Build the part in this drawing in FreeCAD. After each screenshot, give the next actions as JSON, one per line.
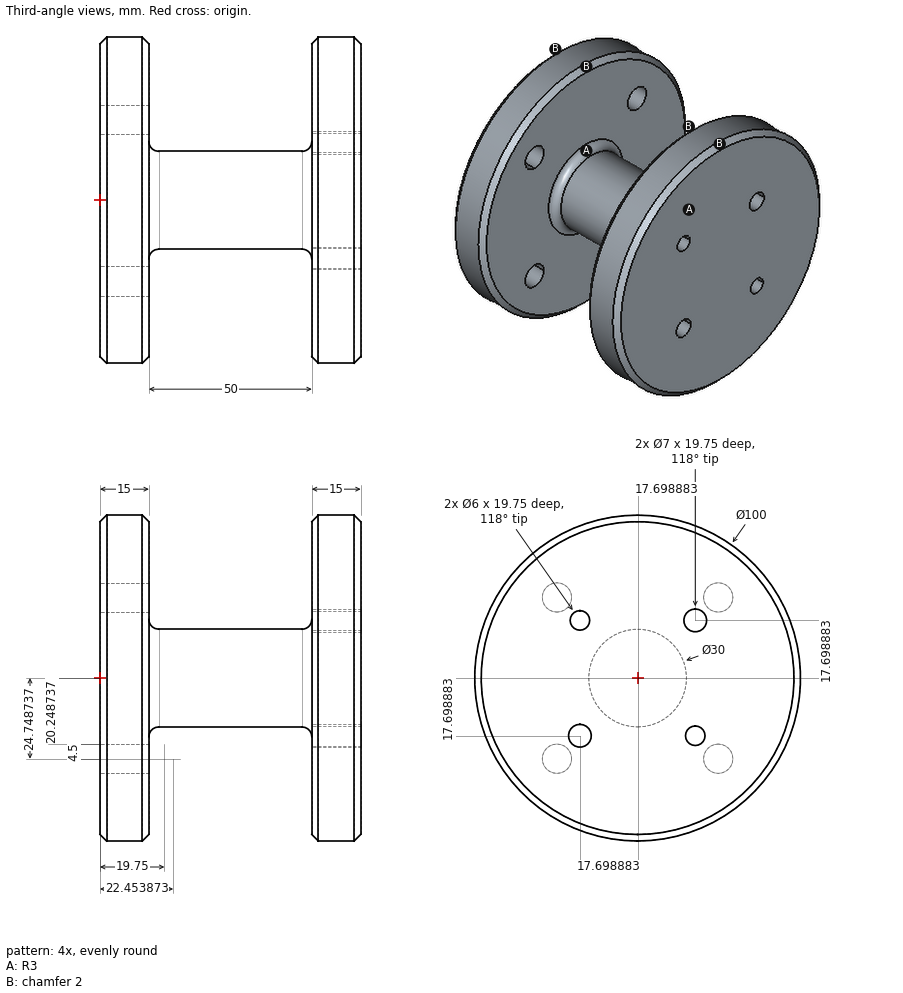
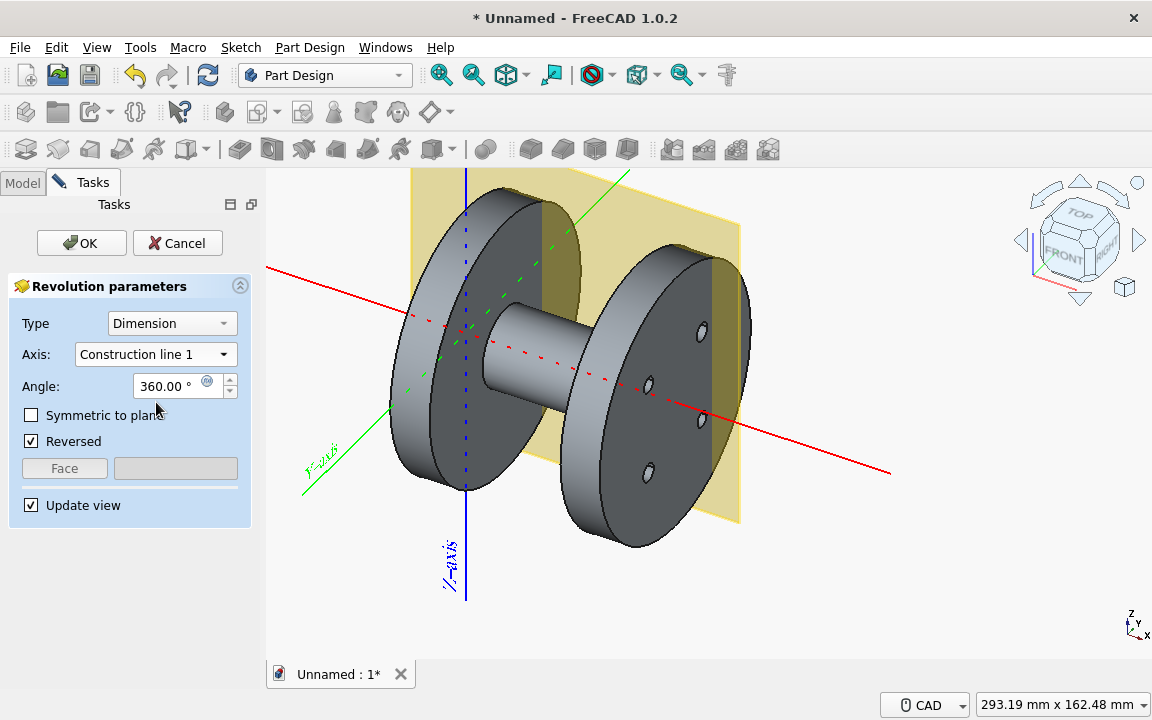
{"action": "left_click", "coordinate": [82, 243]}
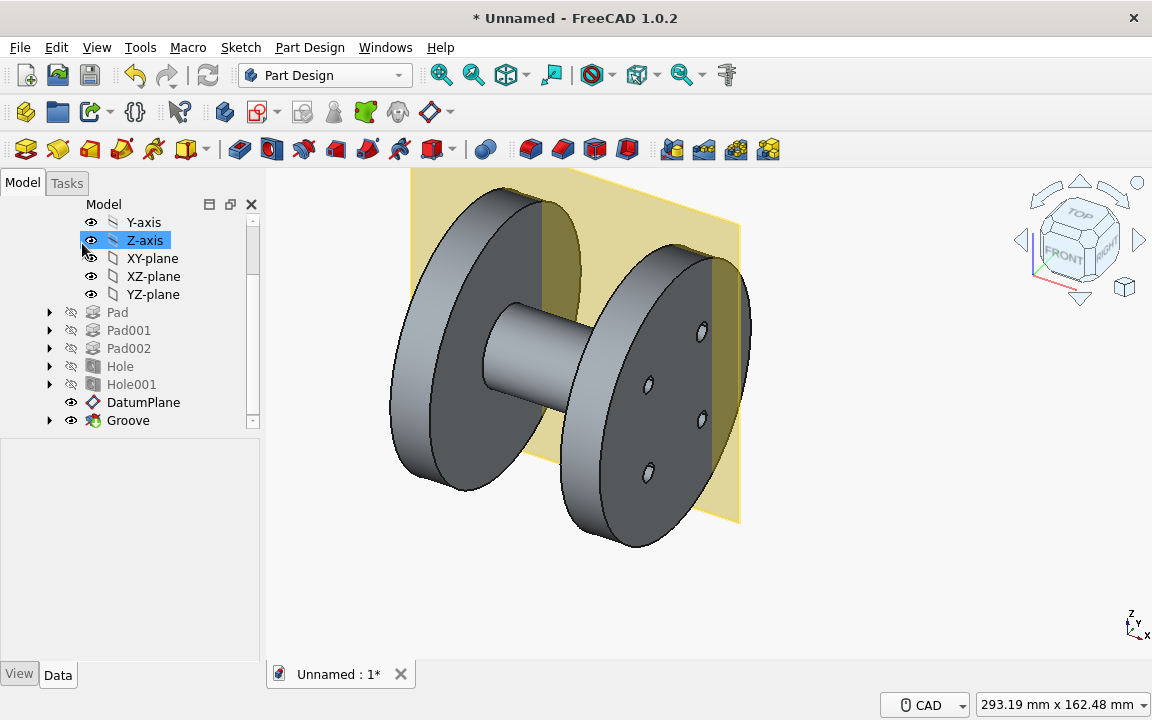
{"action": "left_click", "coordinate": [116, 402]}
{"action": "key", "text": "space"}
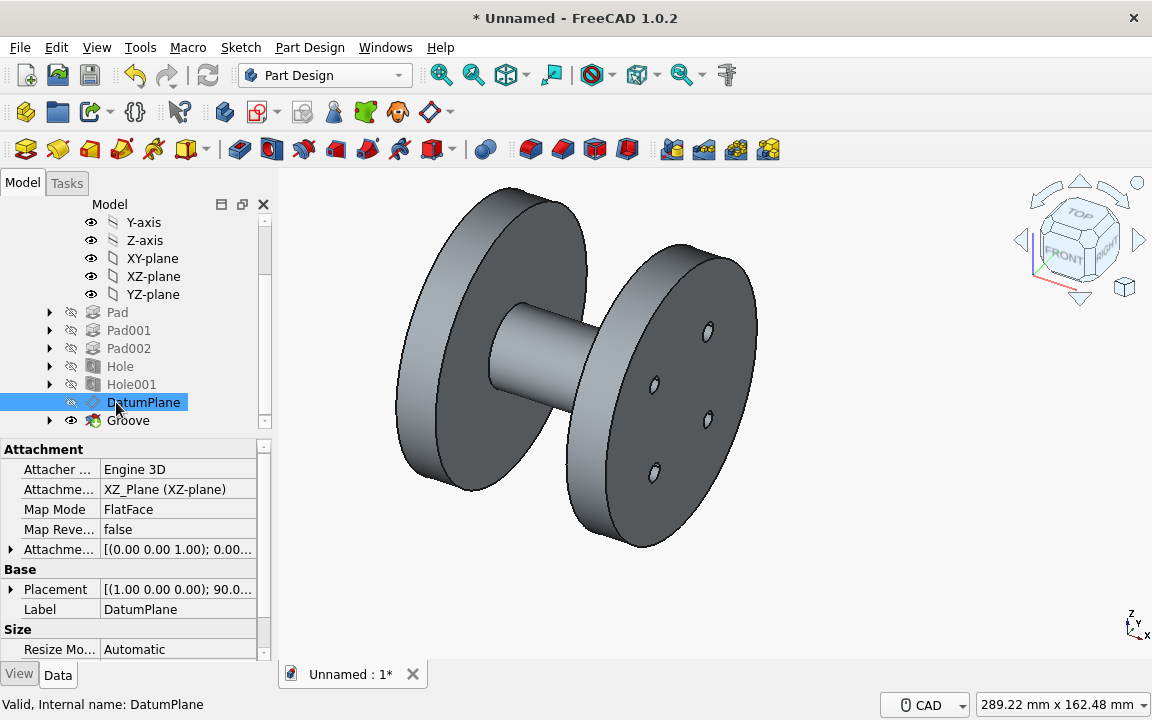
{"action": "left_click", "coordinate": [442, 76]}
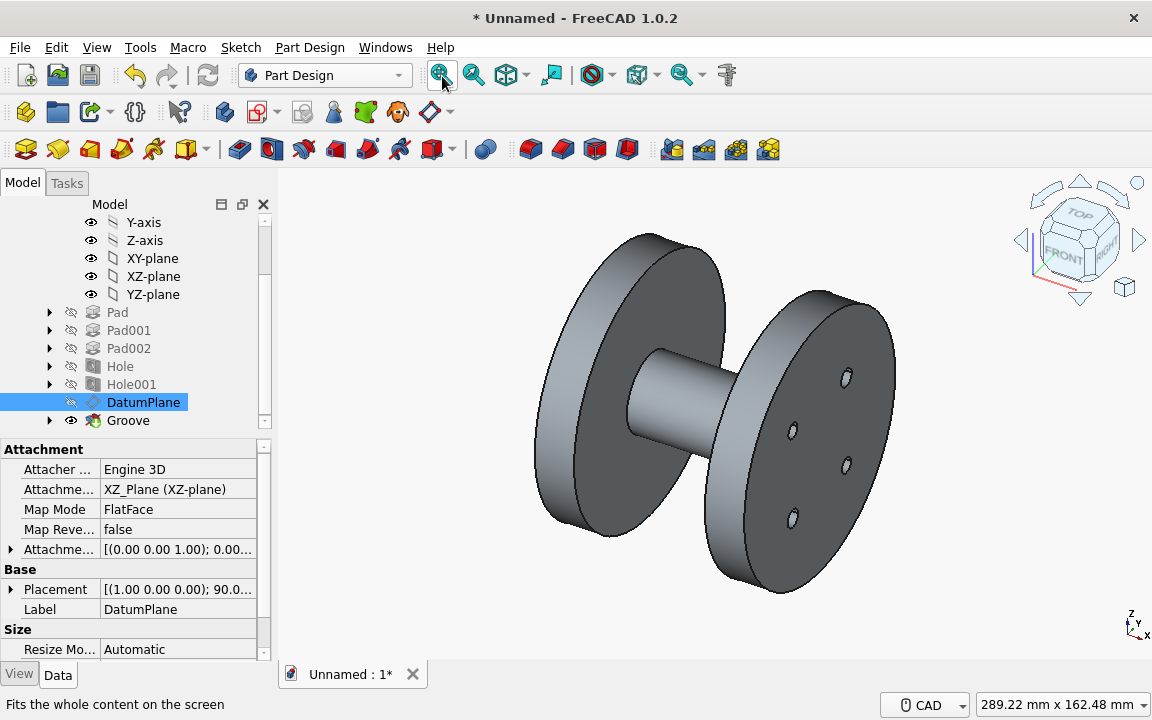
{"action": "left_click", "coordinate": [116, 420]}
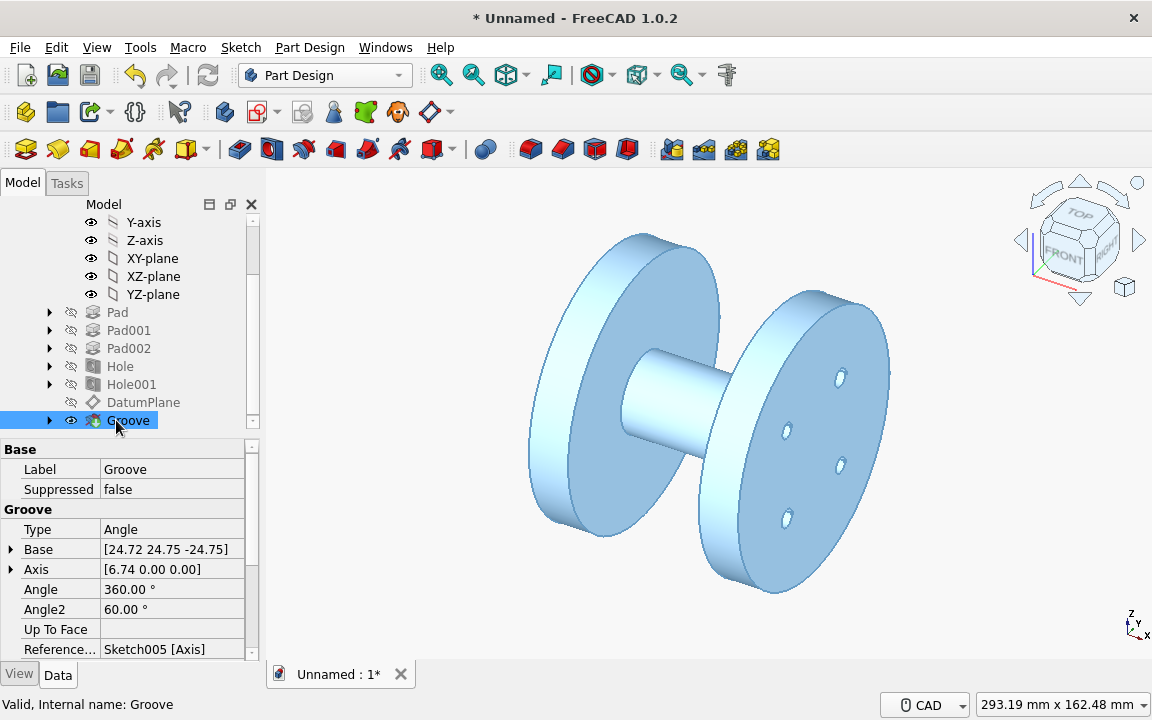
{"action": "left_click", "coordinate": [736, 150]}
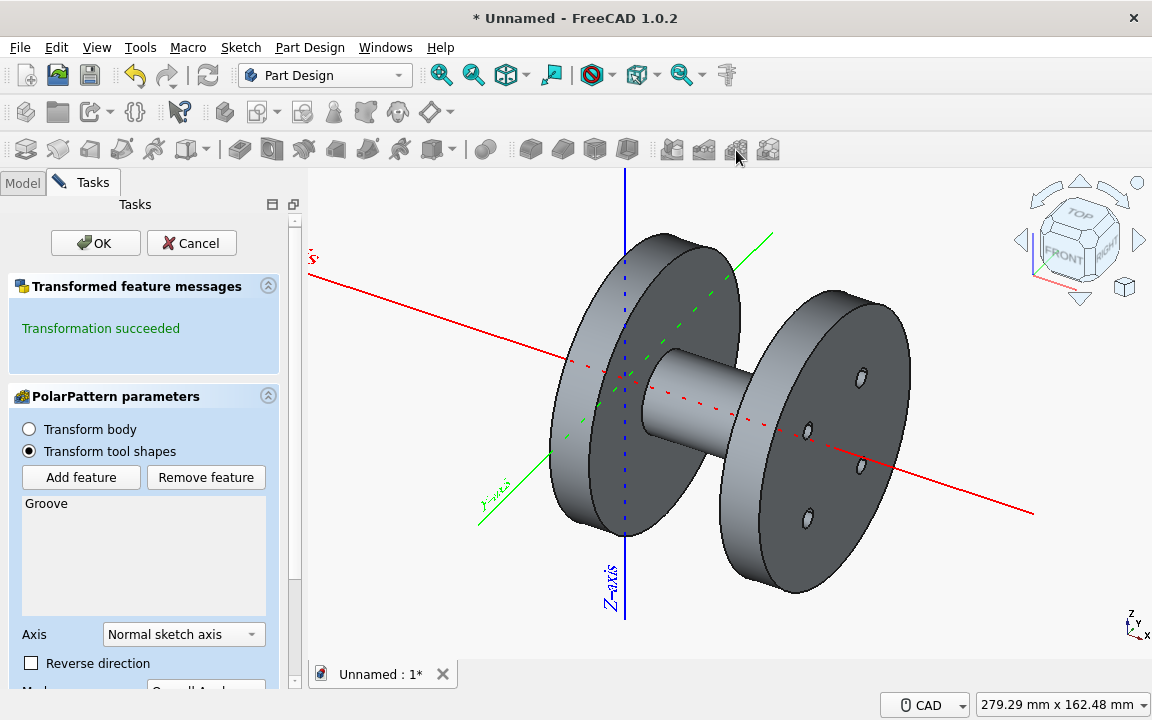
{"action": "left_click", "coordinate": [184, 634]}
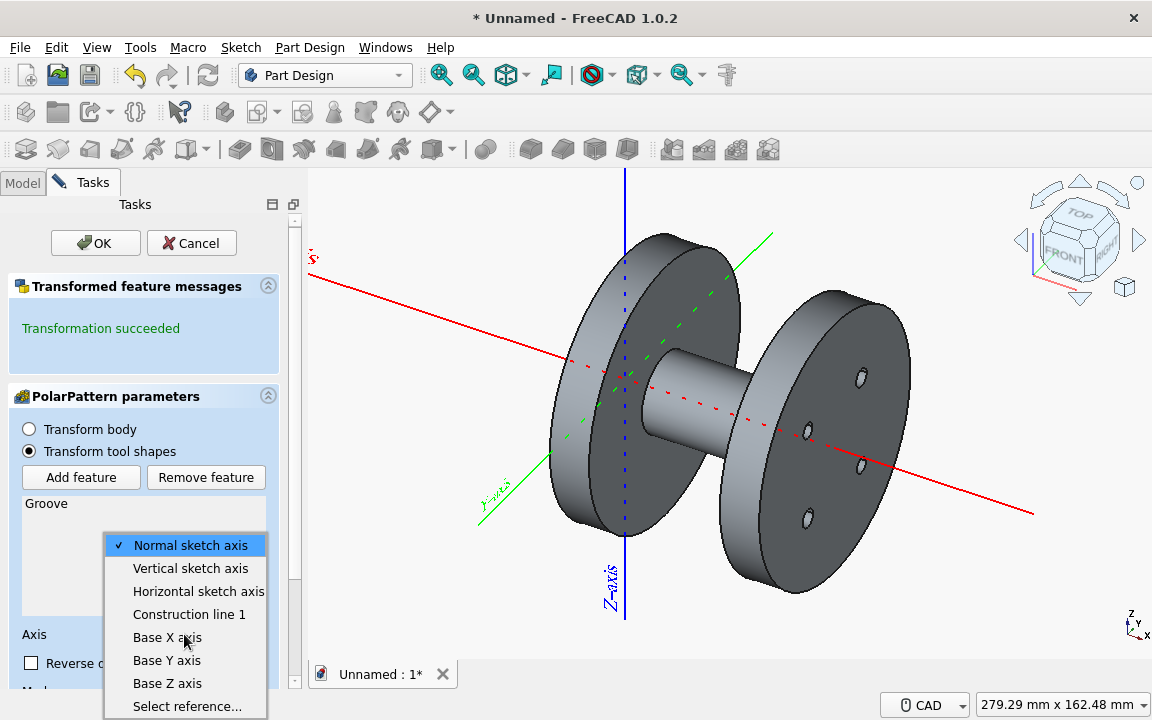
{"action": "left_click", "coordinate": [184, 638]}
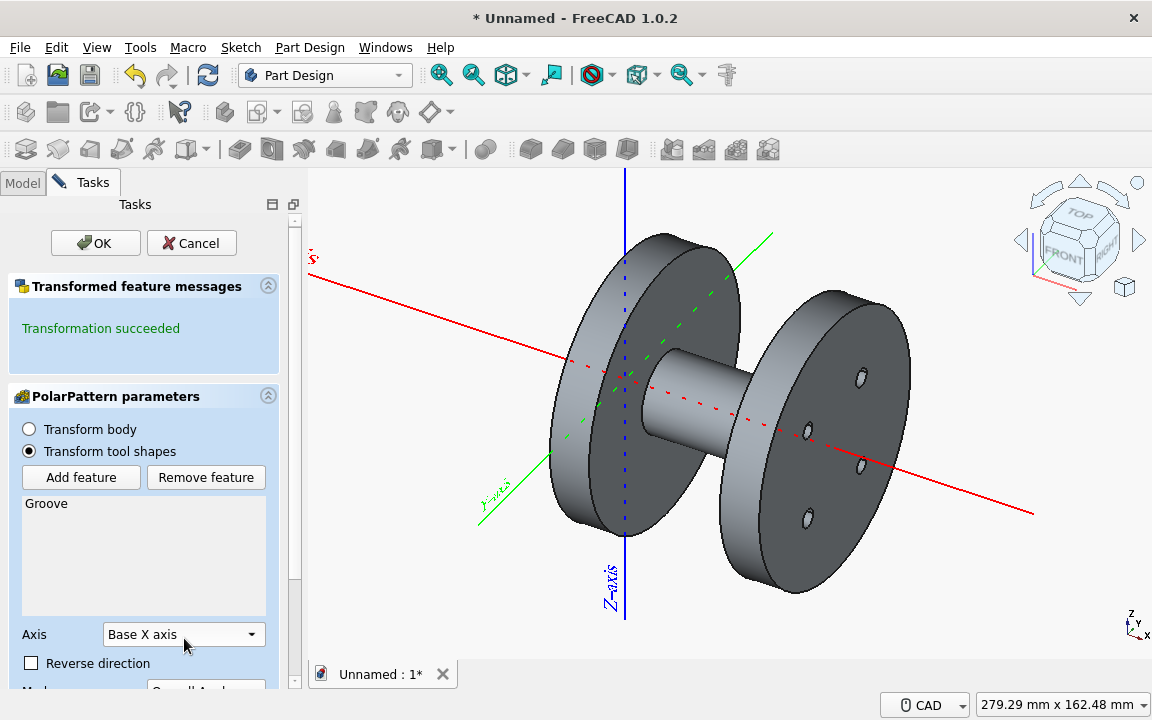
{"action": "scroll", "coordinate": [295, 451], "scroll_direction": "down", "scroll_amount": 3}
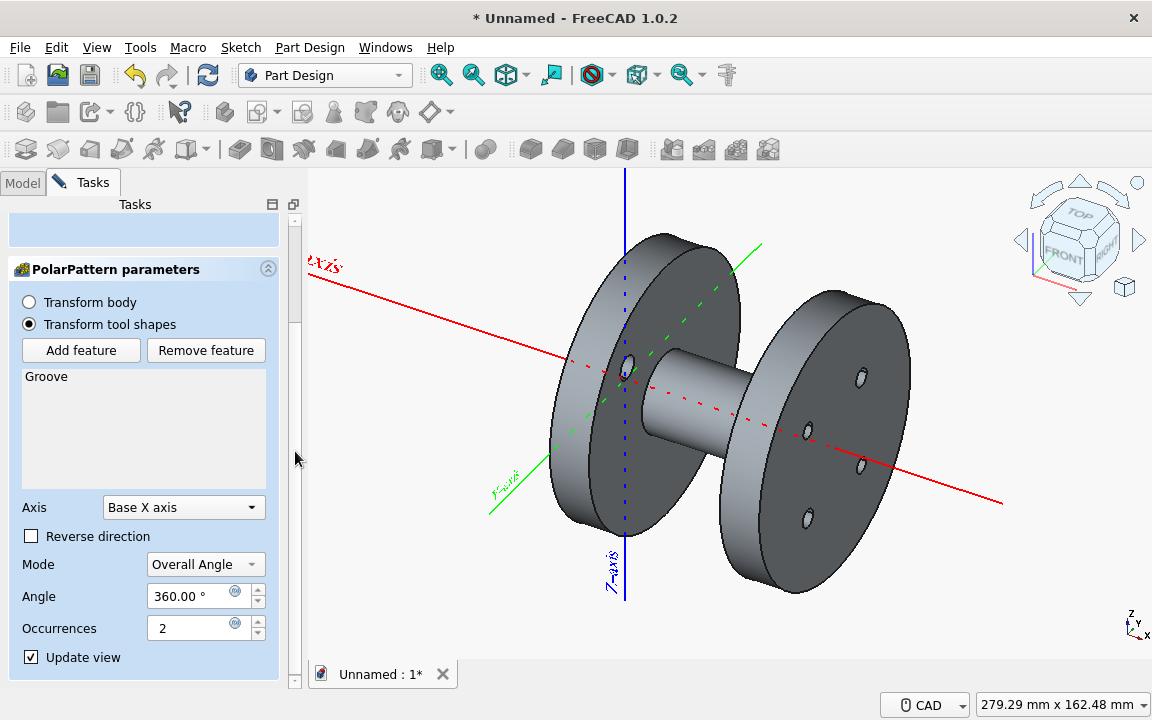
{"action": "triple_click", "coordinate": [198, 628]}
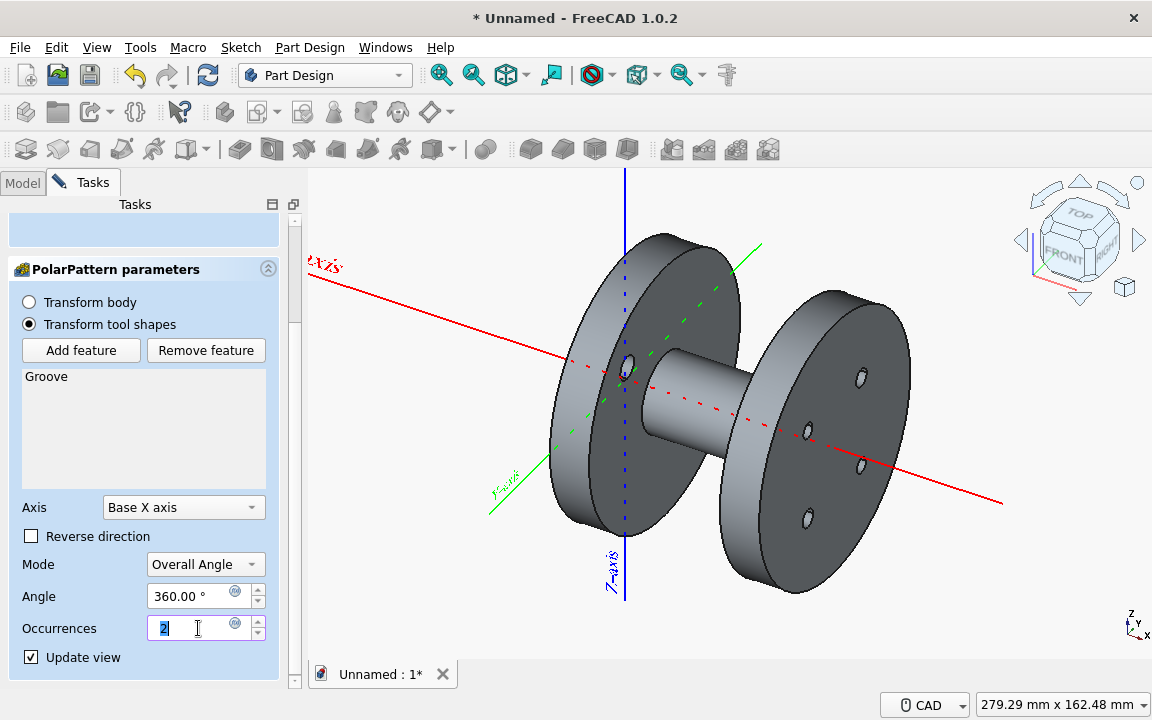
{"action": "type", "text": "4"}
{"action": "key", "text": "Tab"}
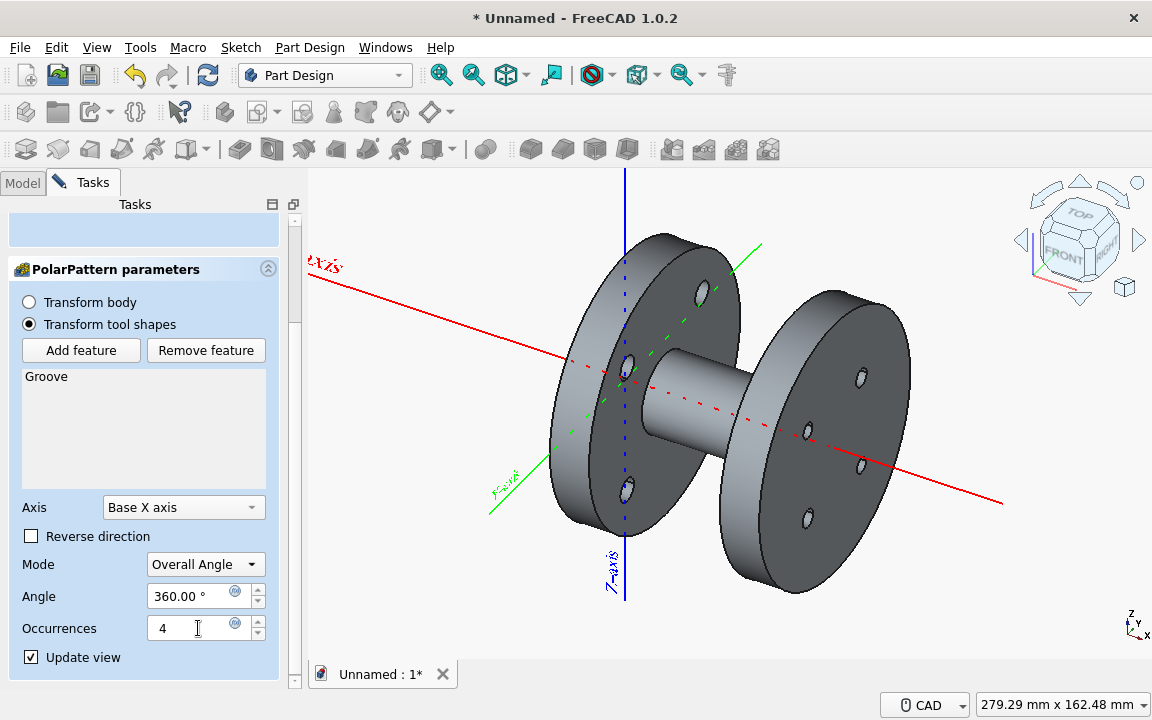
{"action": "scroll", "coordinate": [295, 451], "scroll_direction": "up", "scroll_amount": 3}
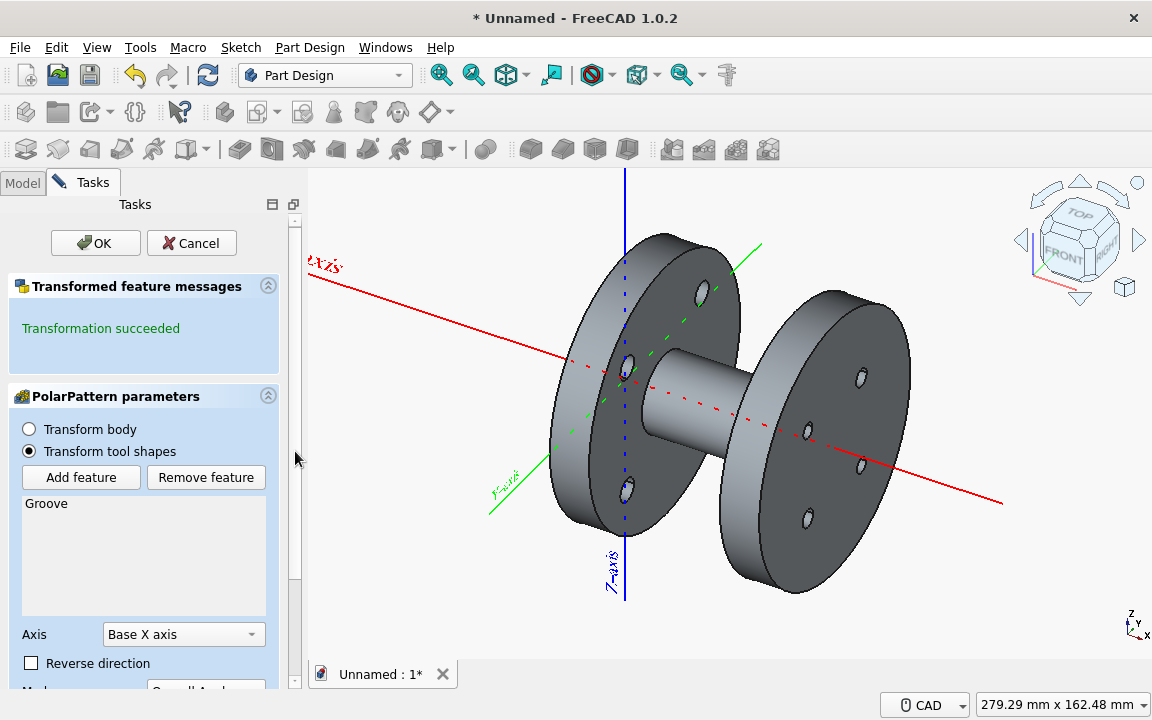
{"action": "left_click", "coordinate": [96, 243]}